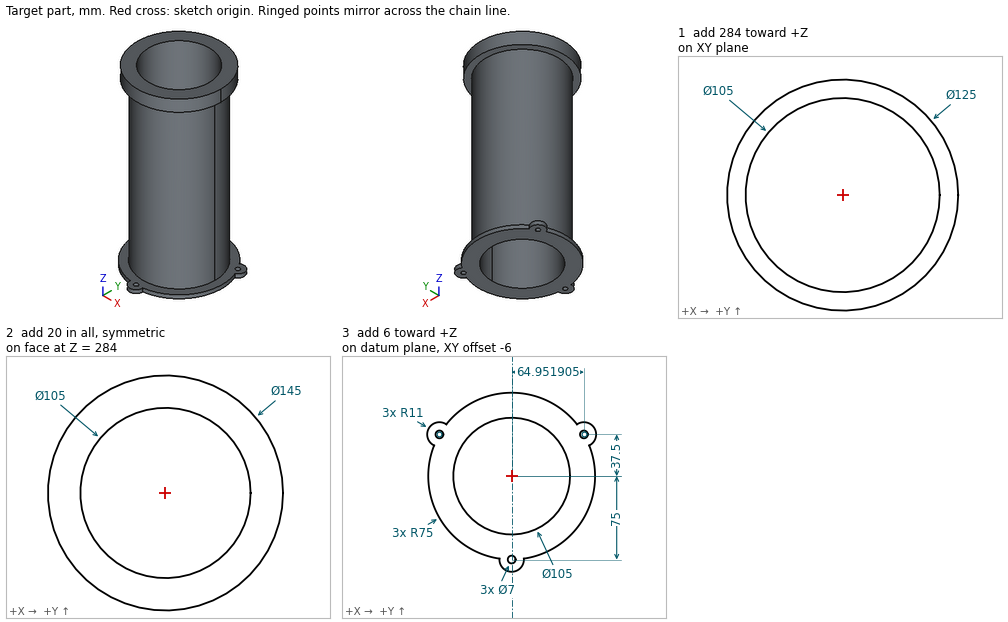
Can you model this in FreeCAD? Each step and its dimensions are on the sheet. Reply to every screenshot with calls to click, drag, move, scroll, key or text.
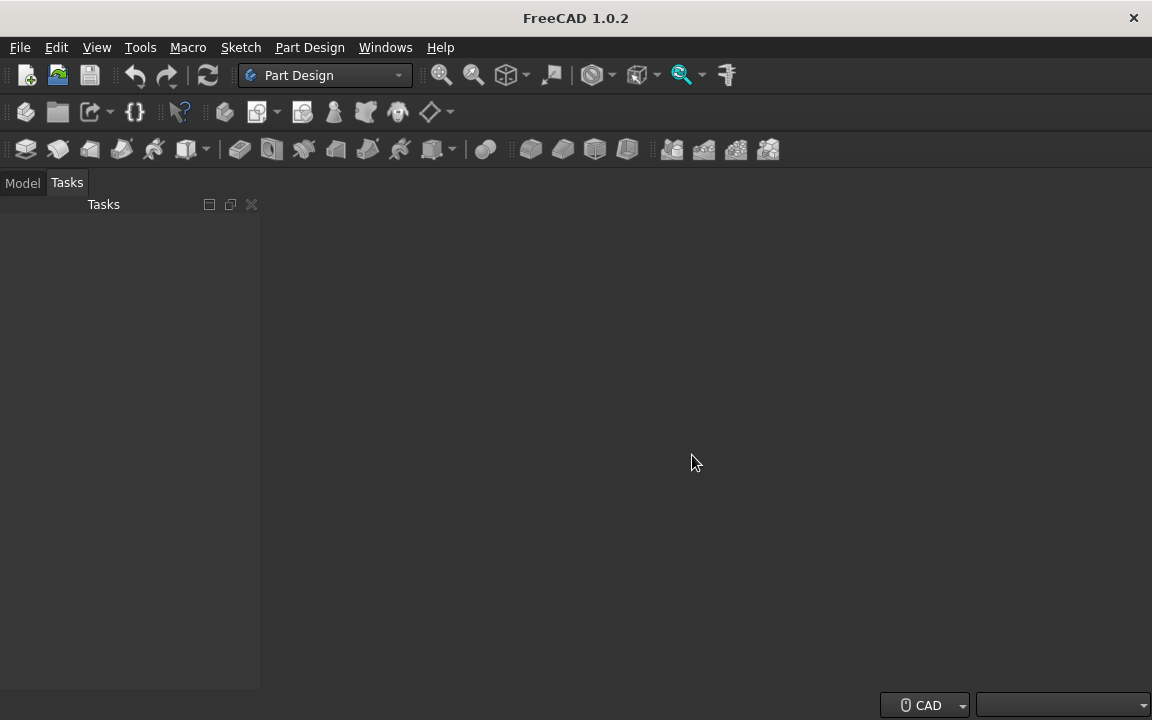
key(ctrl+n)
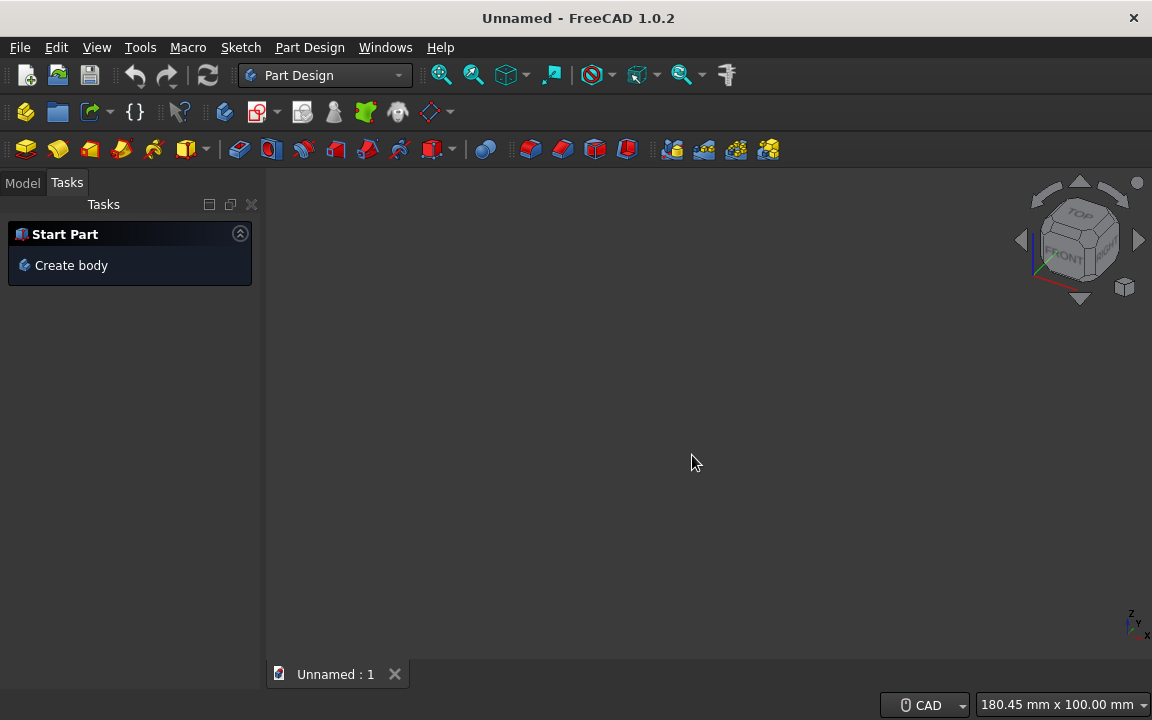
click(258, 112)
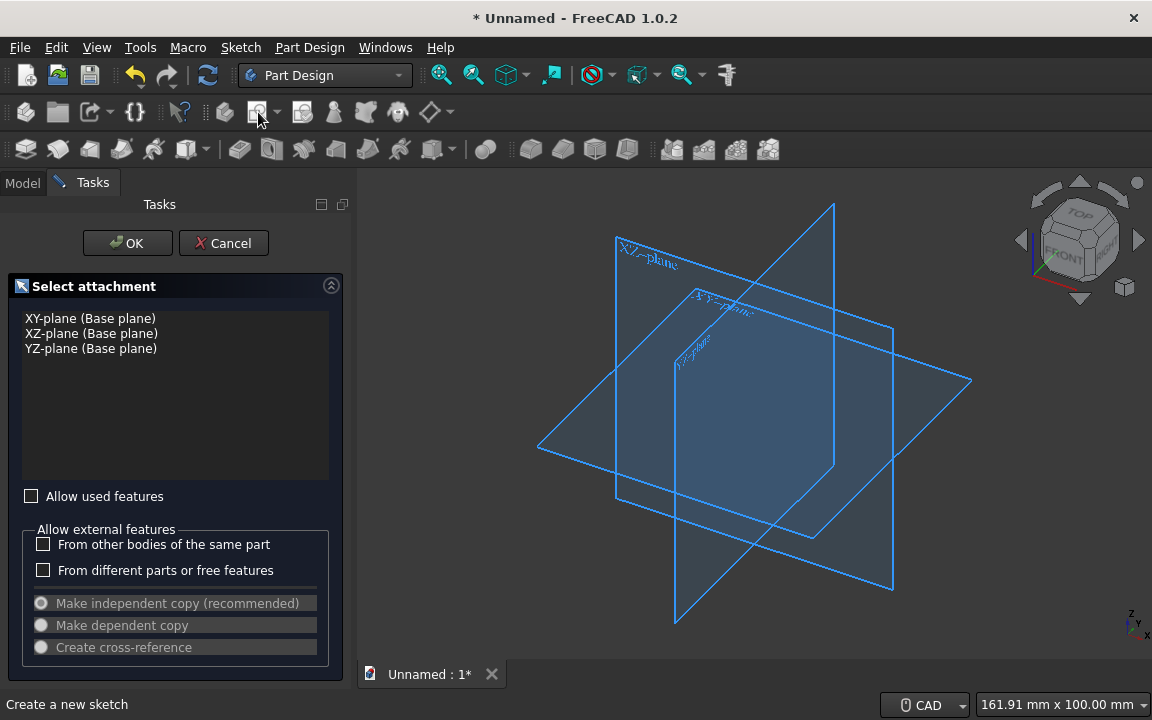
click(82, 318)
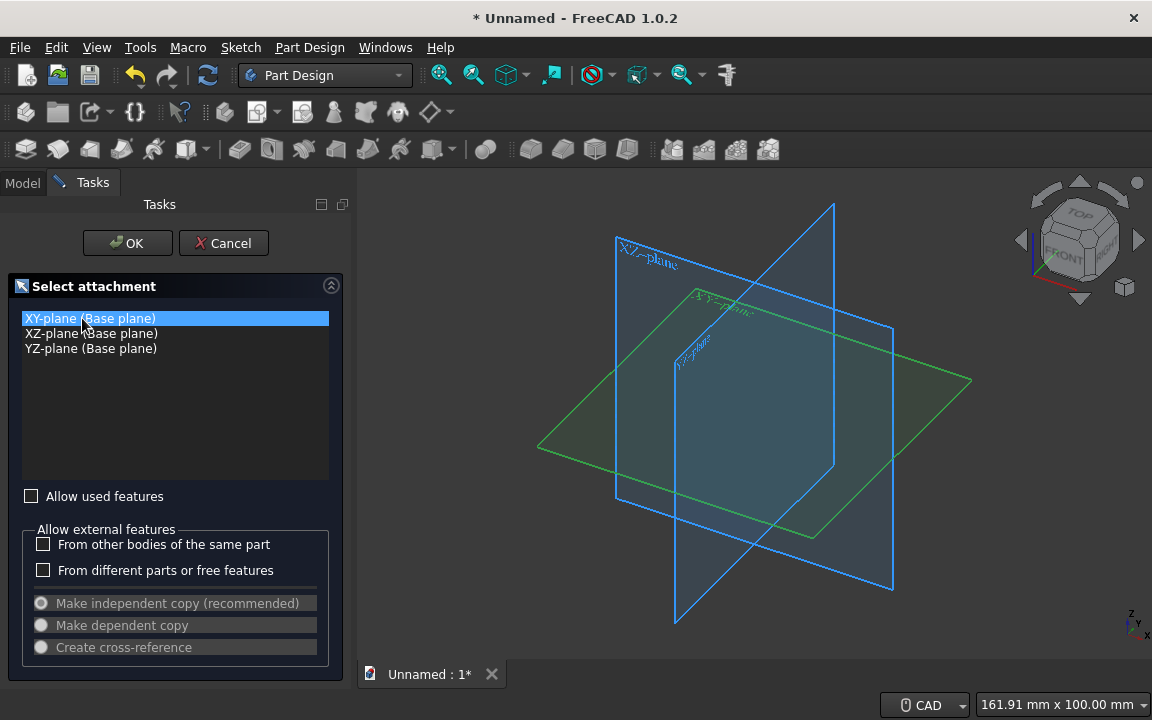
click(128, 243)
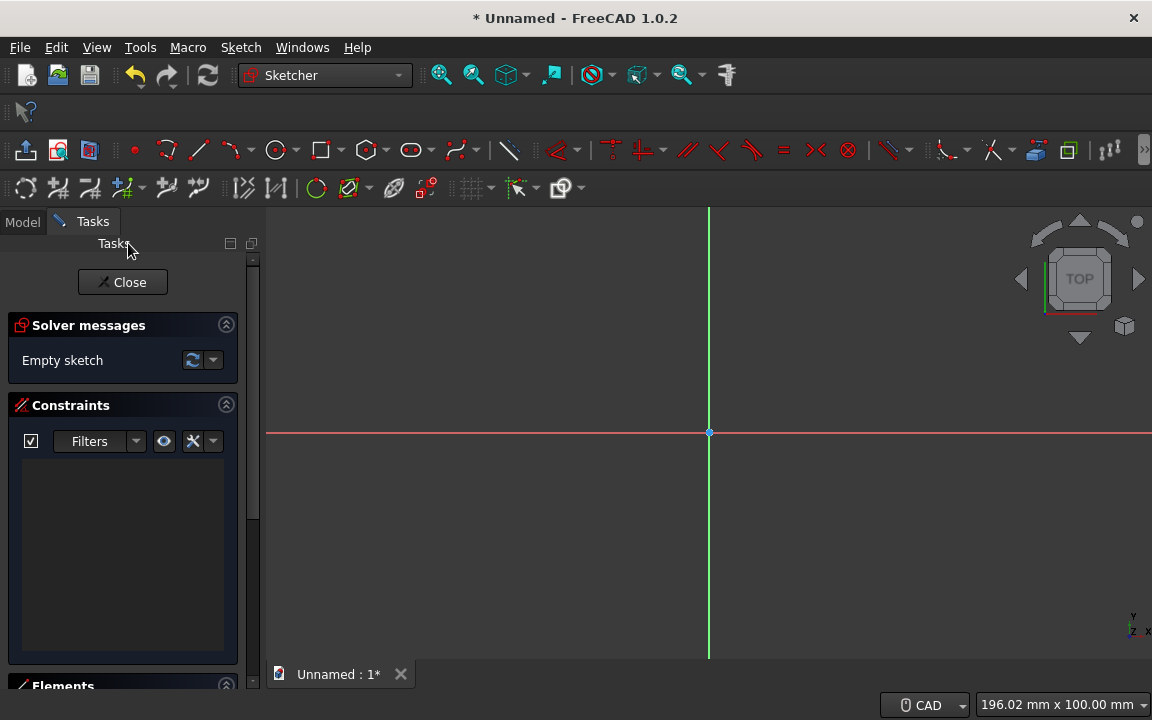
scroll(585, 433, down, 4)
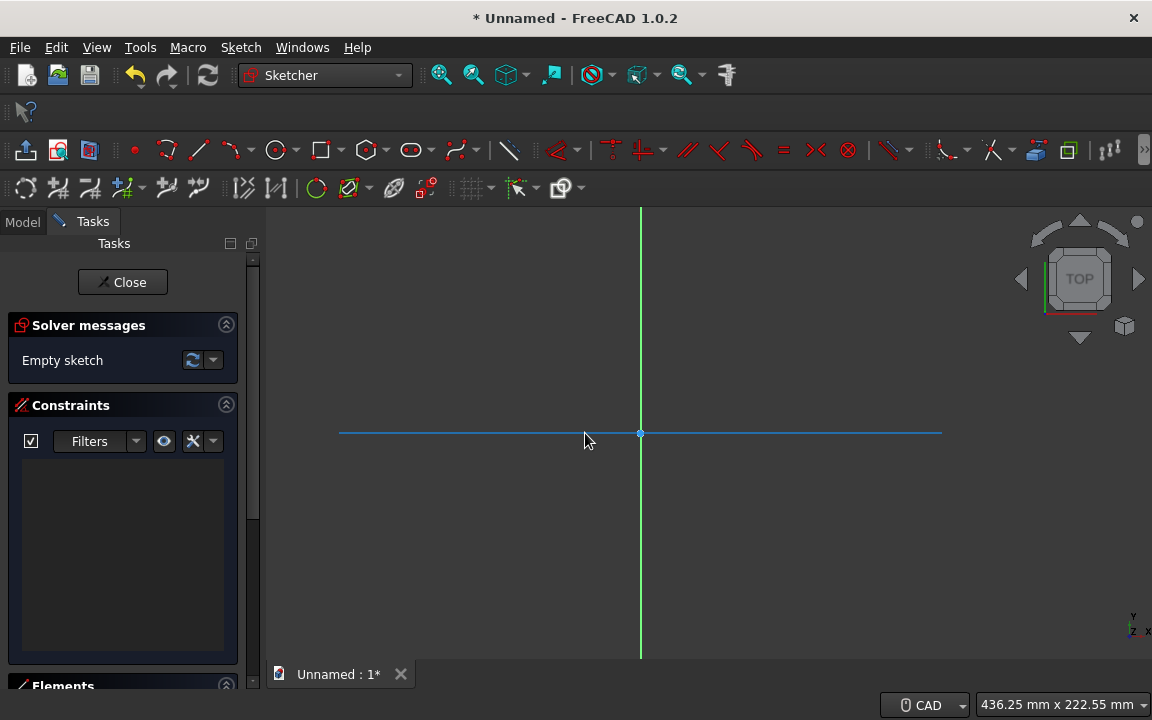
click(276, 150)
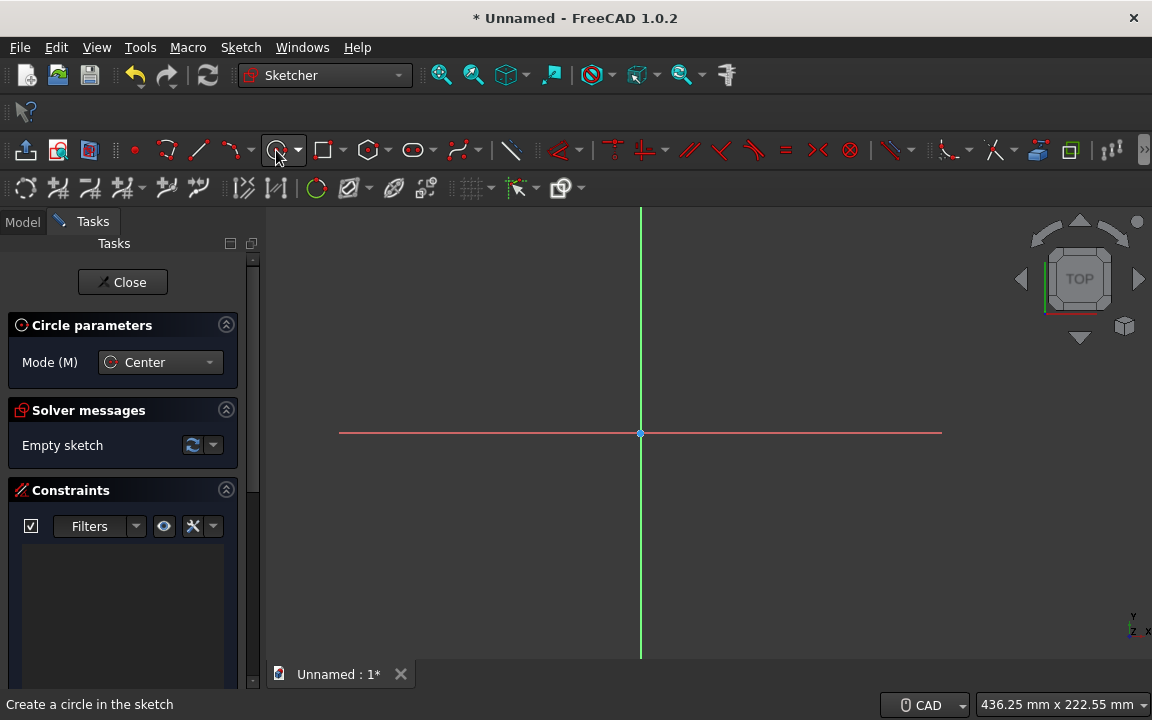
click(641, 433)
click(731, 344)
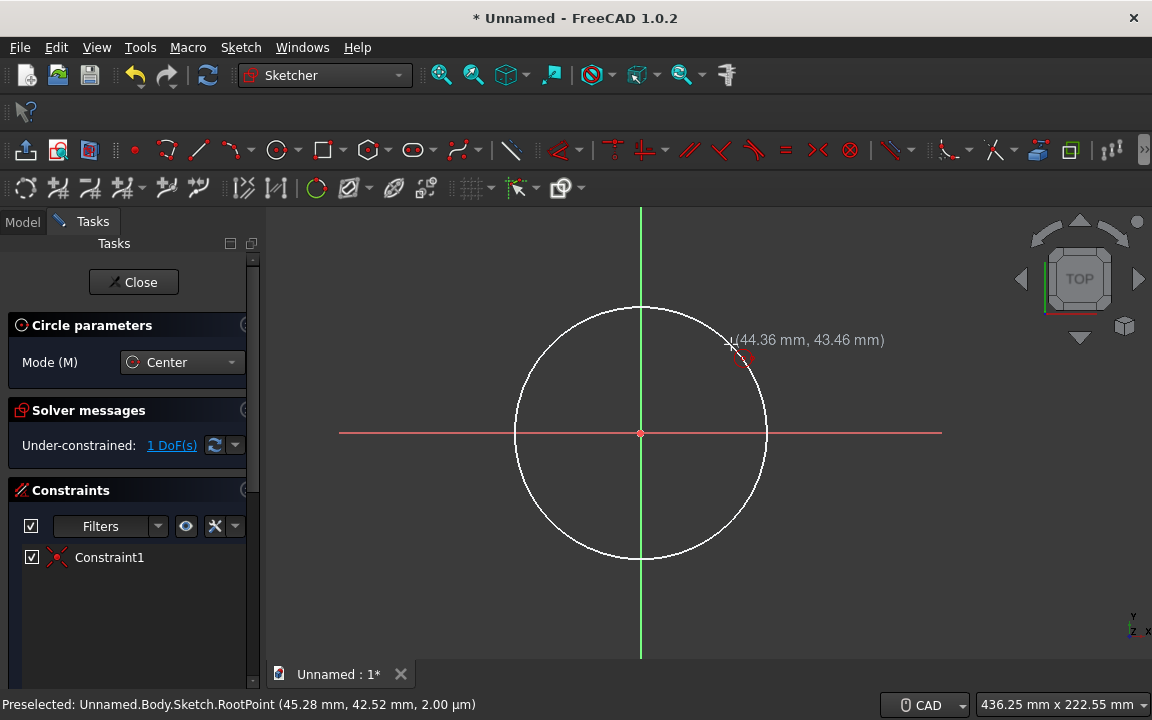
click(641, 433)
click(716, 358)
key(Escape)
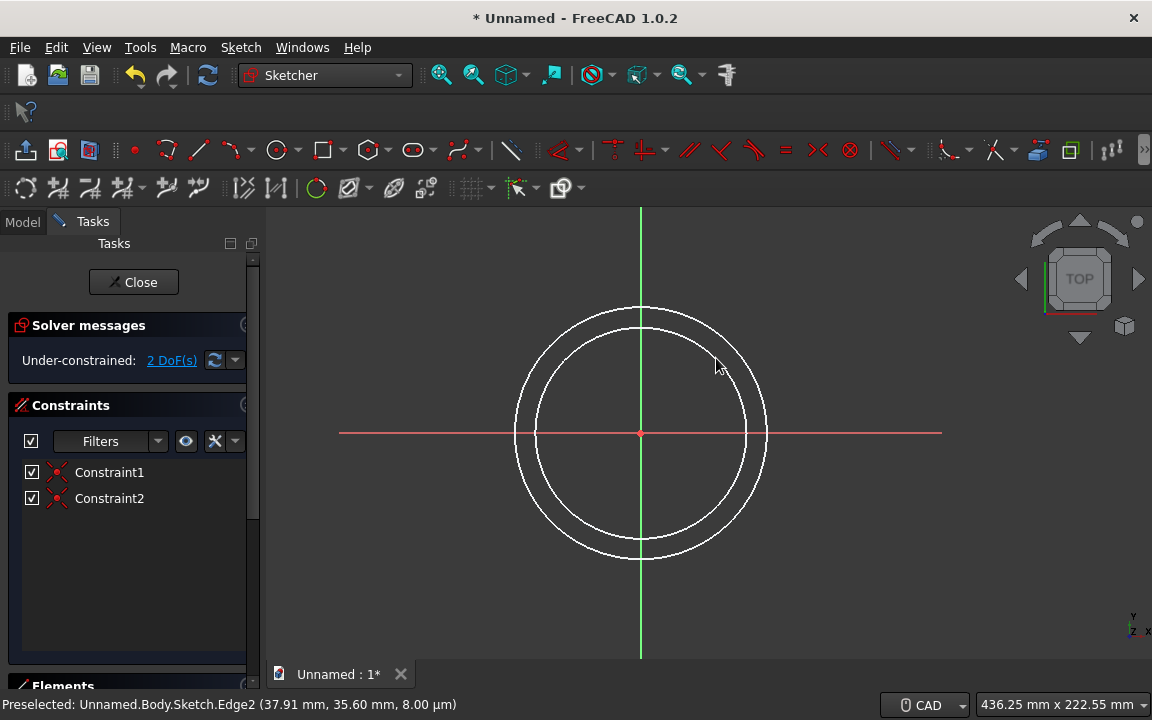
click(558, 150)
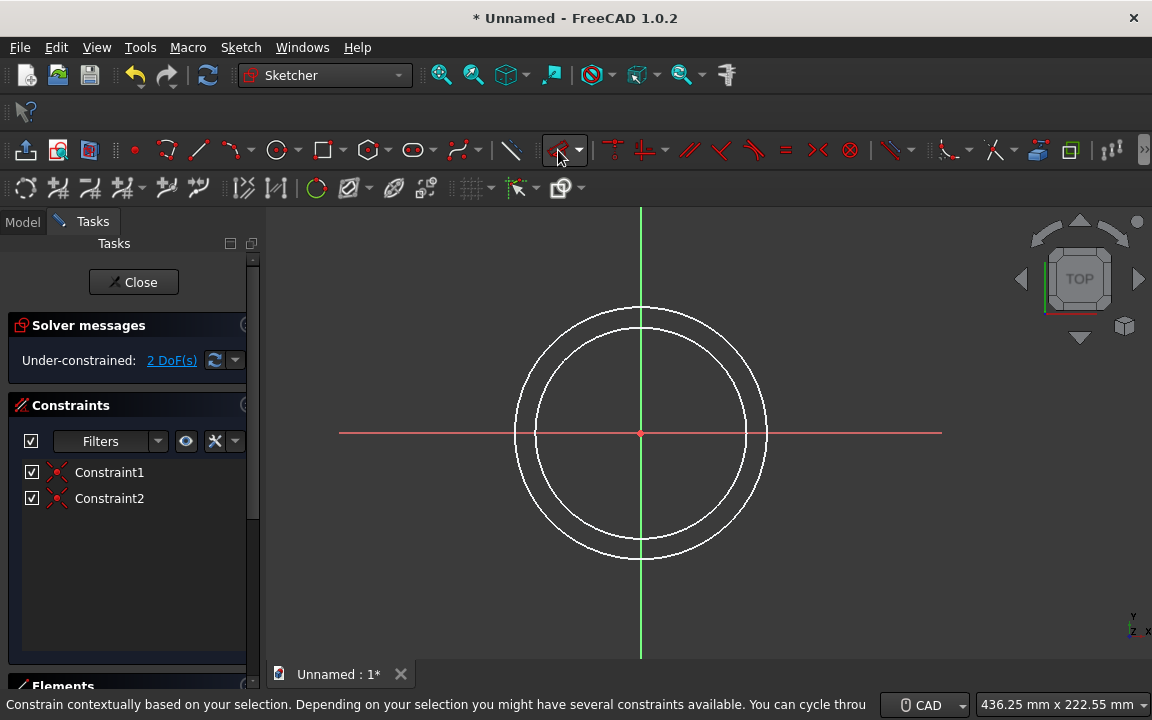
click(730, 344)
click(753, 321)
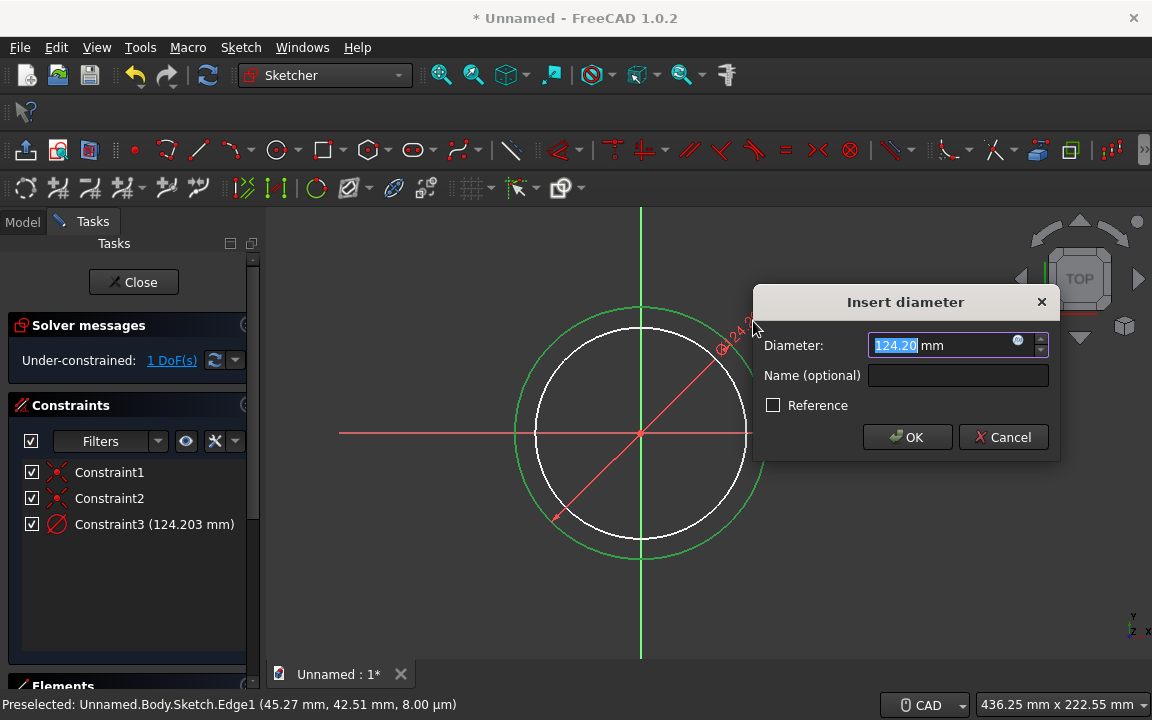
text(125)
key(Return)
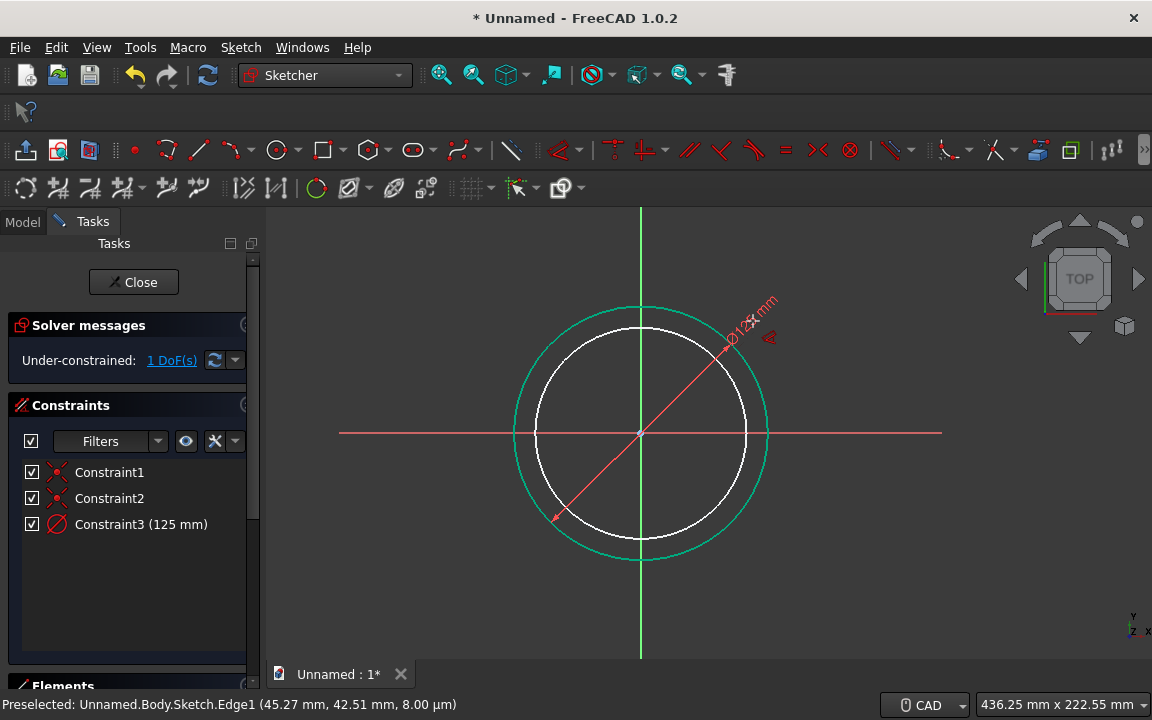
click(715, 358)
click(795, 387)